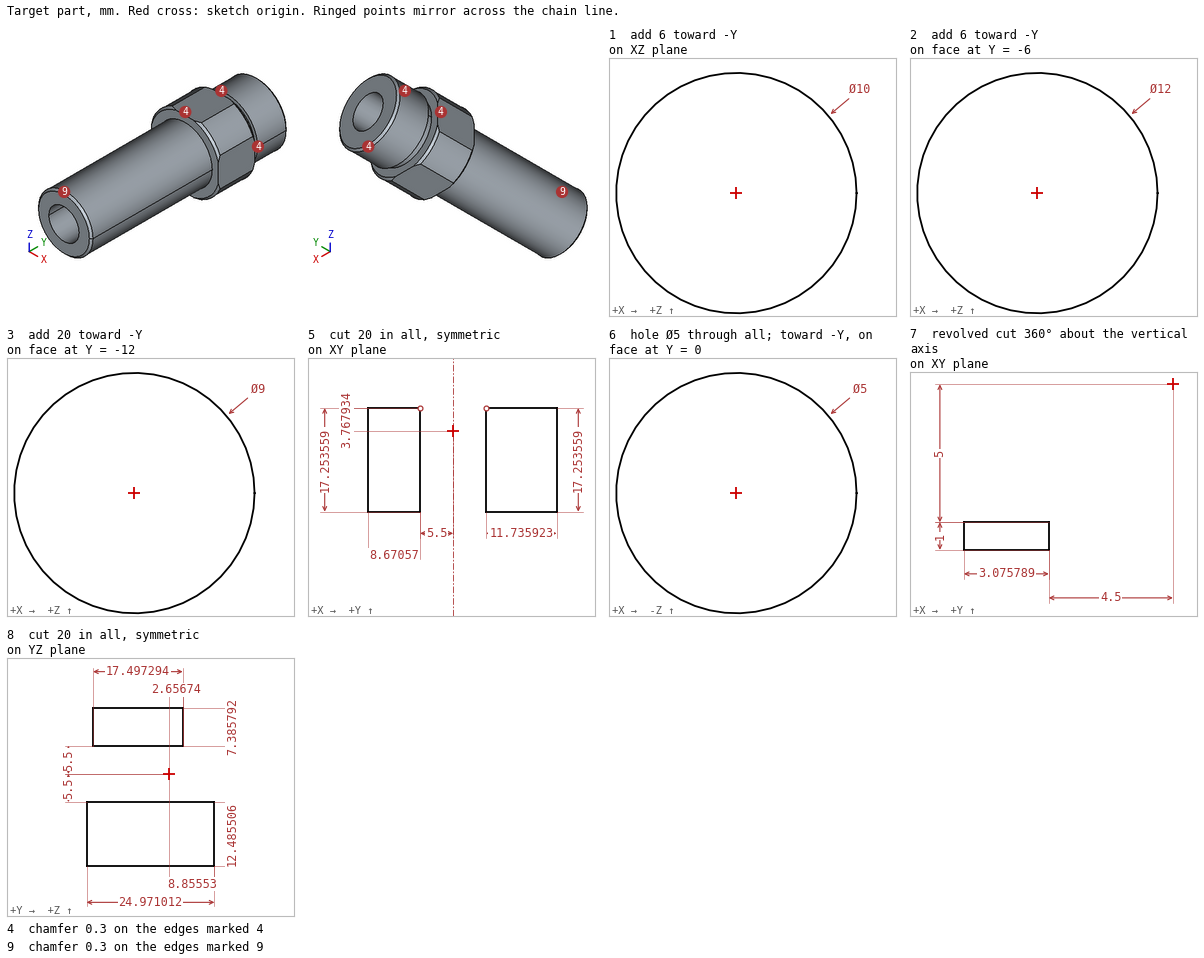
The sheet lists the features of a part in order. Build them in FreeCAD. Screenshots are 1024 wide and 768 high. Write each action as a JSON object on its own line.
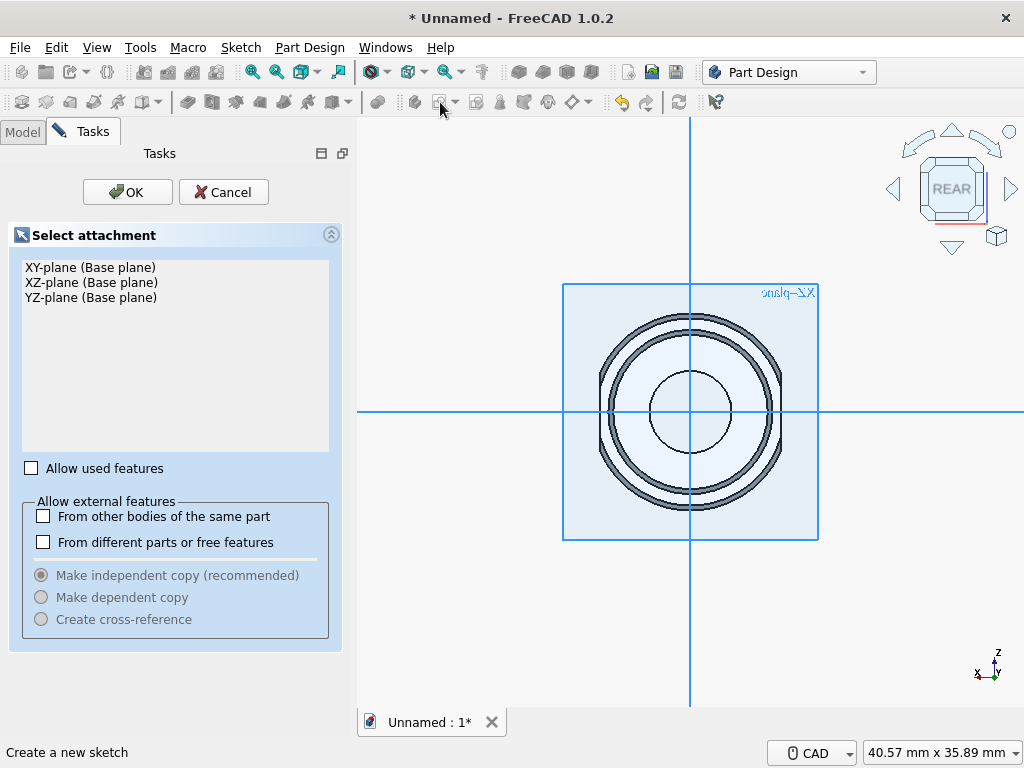
{"action": "left_click", "coordinate": [82, 268]}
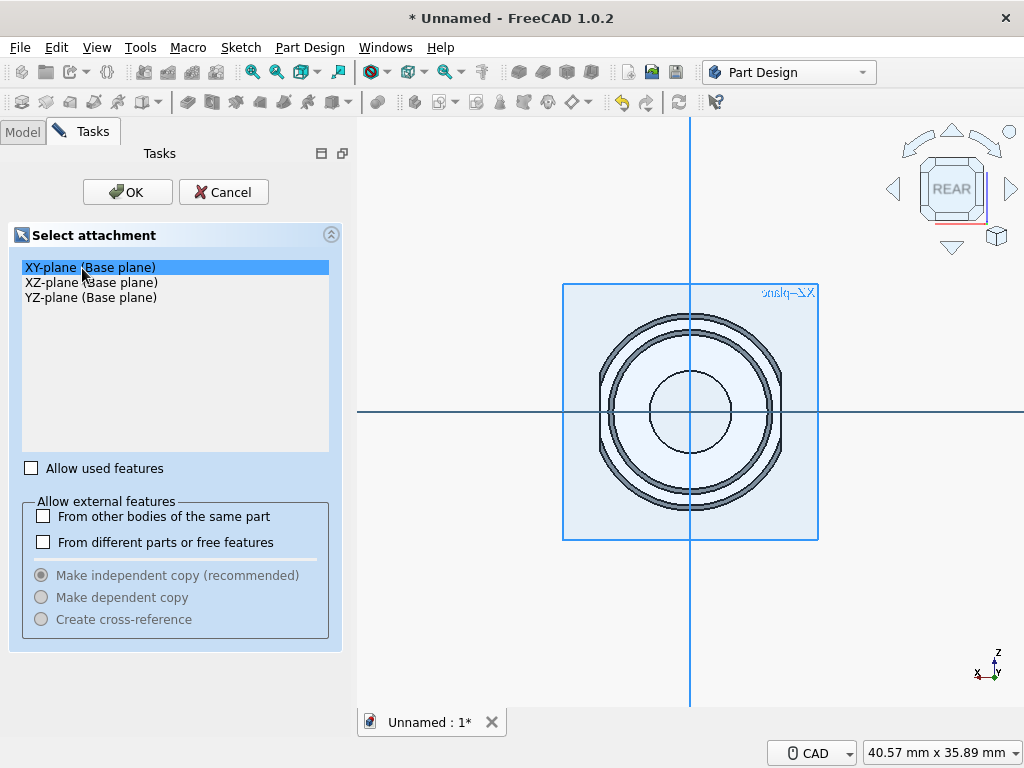
{"action": "left_click", "coordinate": [128, 192]}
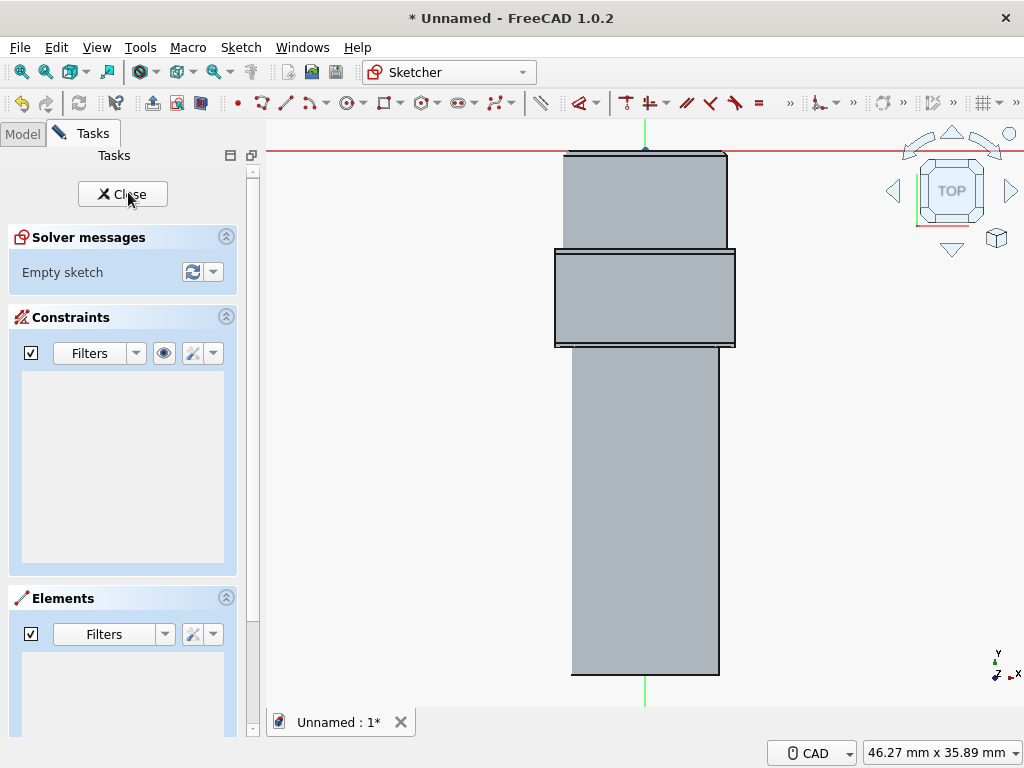
{"action": "left_click", "coordinate": [202, 104]}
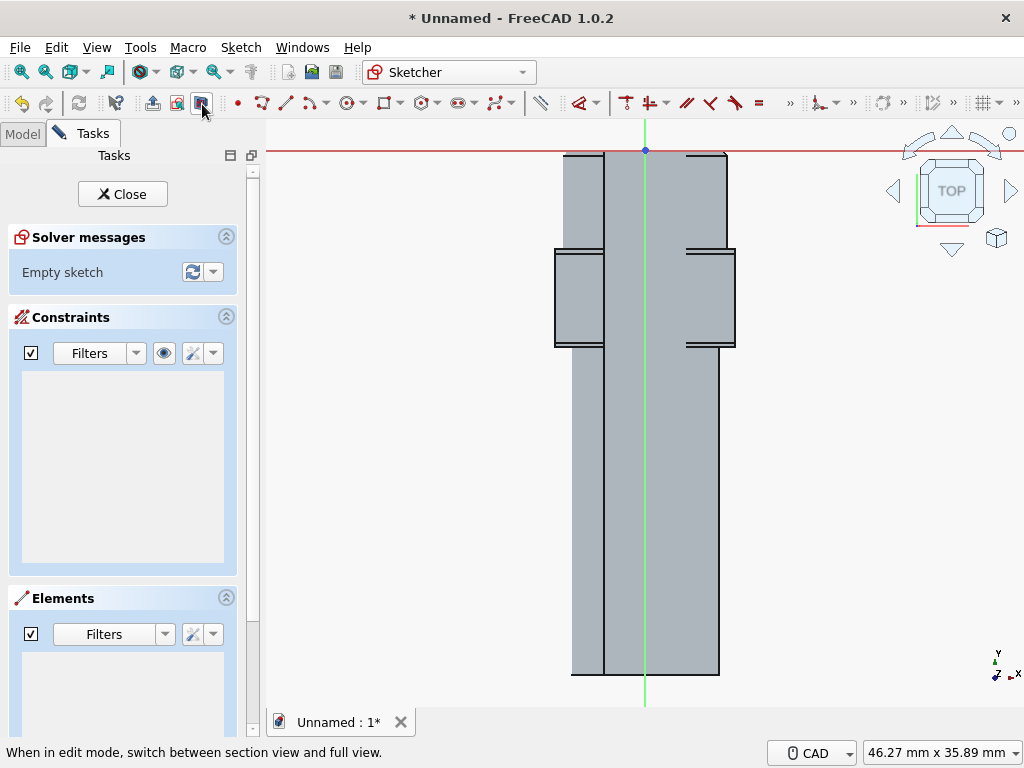
{"action": "scroll", "coordinate": [576, 413], "scroll_direction": "down", "scroll_amount": 5}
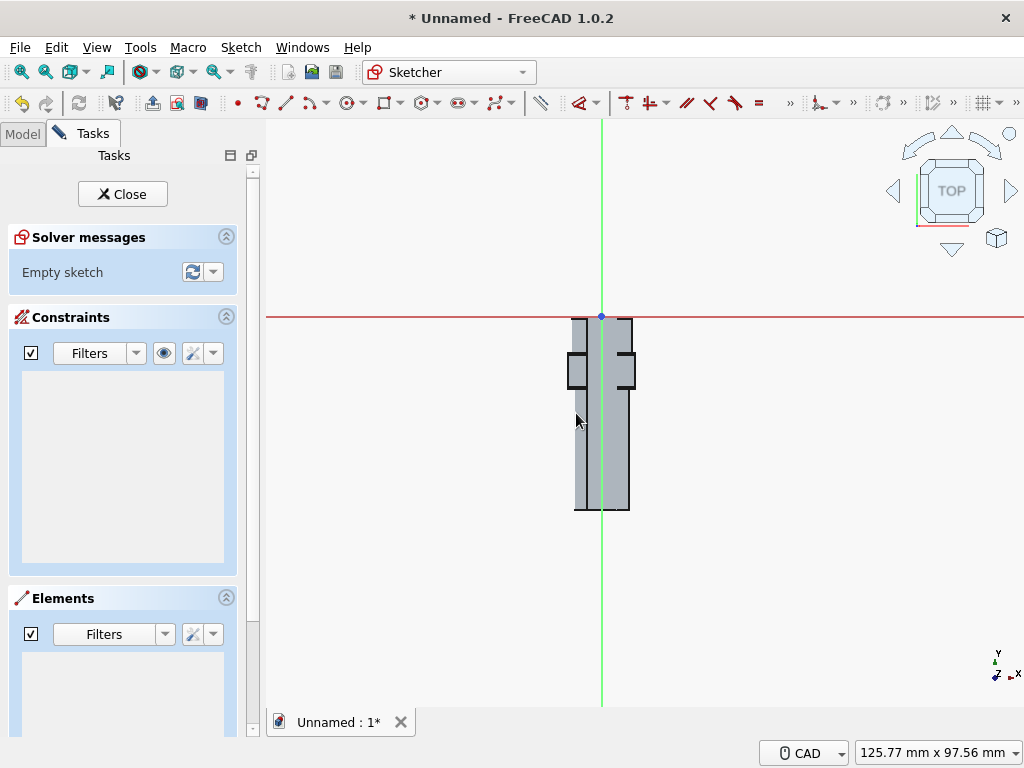
{"action": "scroll", "coordinate": [579, 325], "scroll_direction": "up", "scroll_amount": 11}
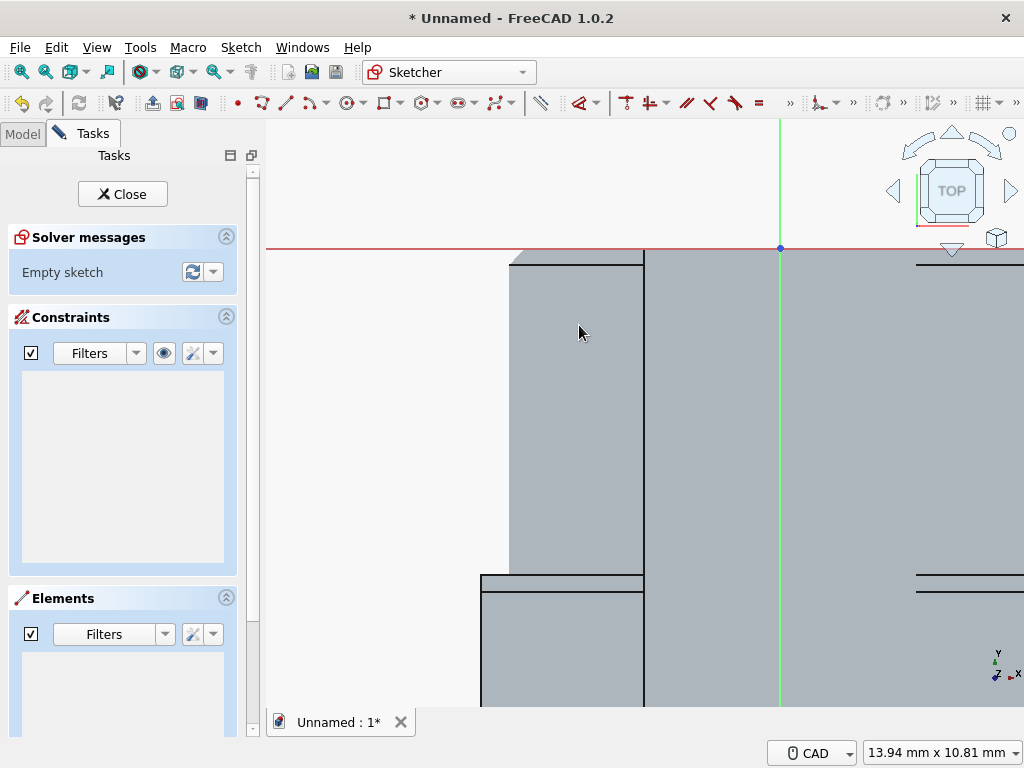
{"action": "key", "text": "g r"}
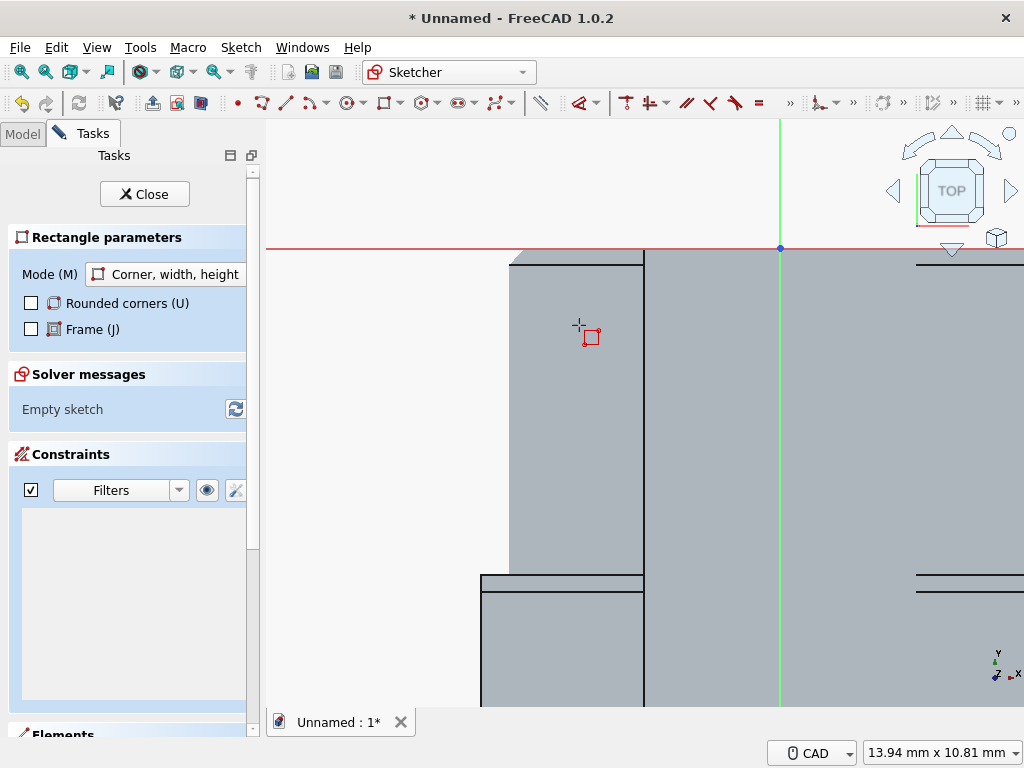
{"action": "left_click", "coordinate": [368, 521]}
{"action": "mouse_move", "coordinate": [535, 575]}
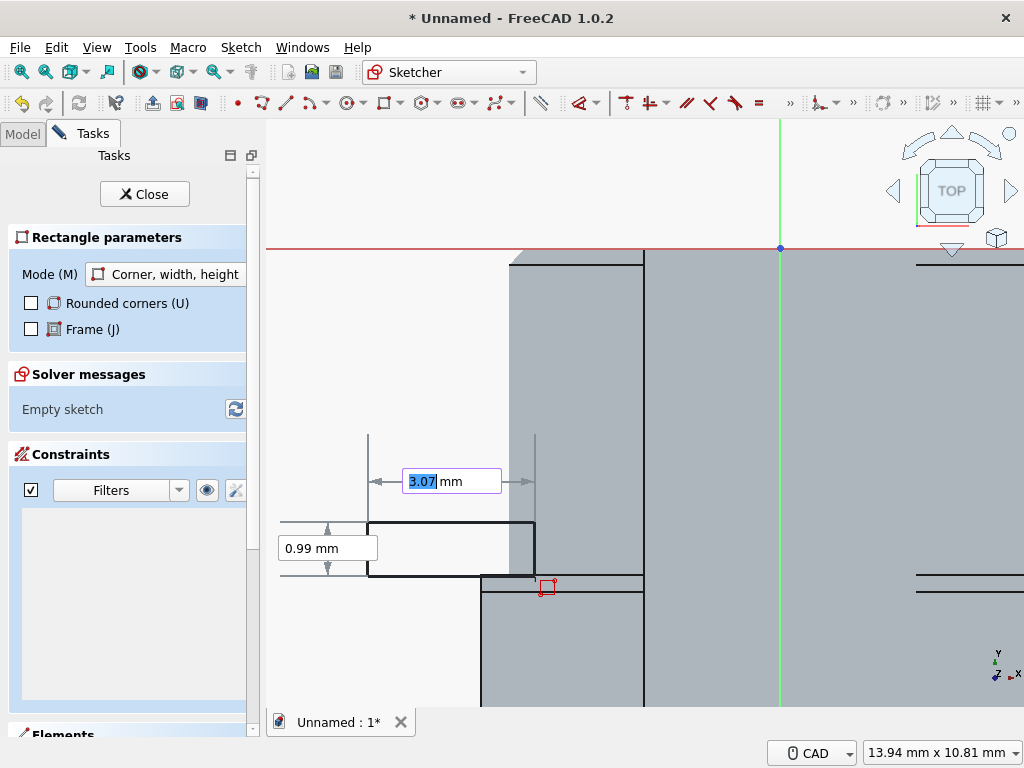
{"action": "type", "text": "3.075789"}
{"action": "key", "text": "Tab"}
{"action": "type", "text": "1"}
{"action": "key", "text": "Return"}
{"action": "key", "text": "Escape"}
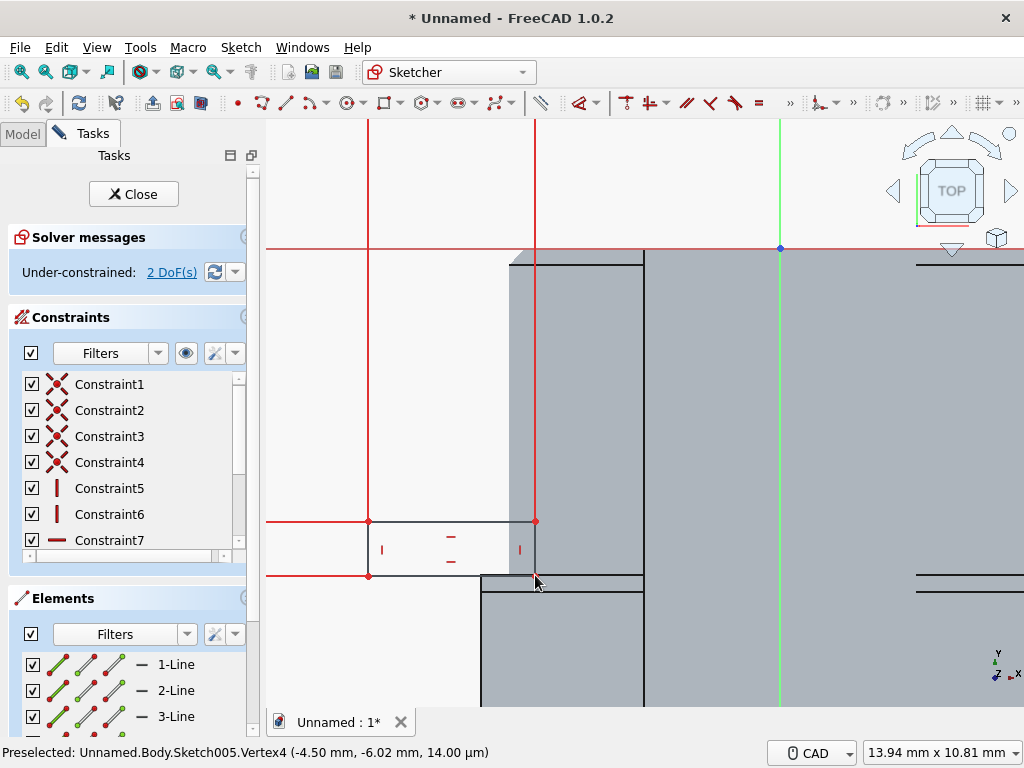
{"action": "key", "text": "d"}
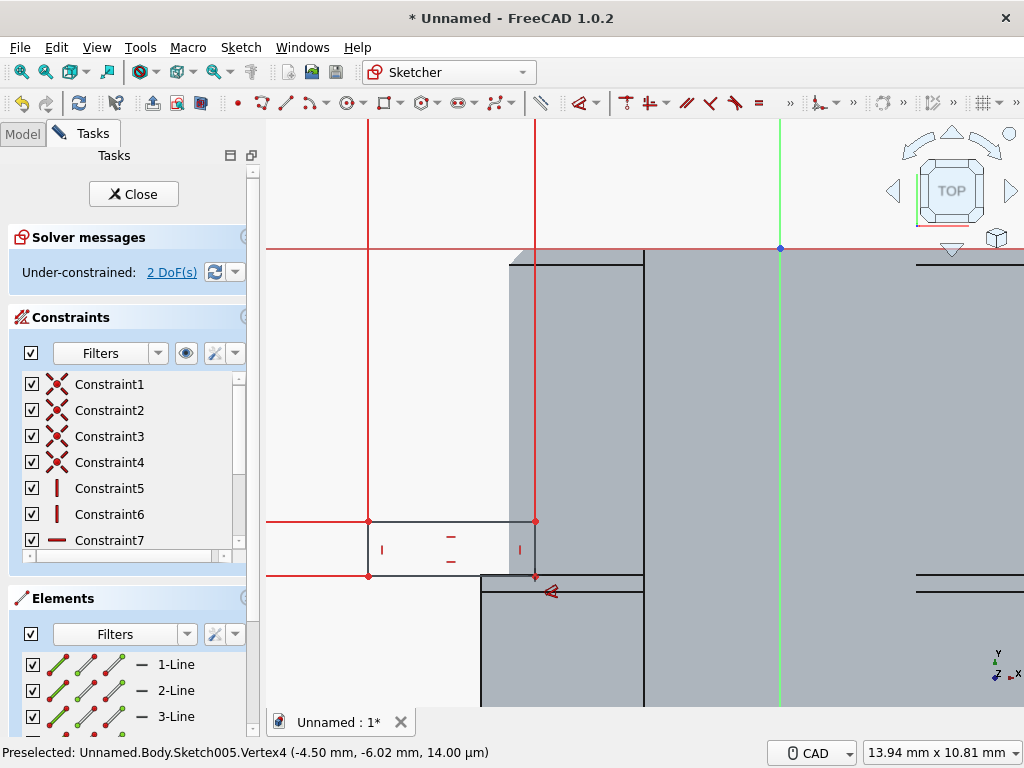
{"action": "left_click", "coordinate": [368, 522]}
{"action": "left_click", "coordinate": [814, 385]}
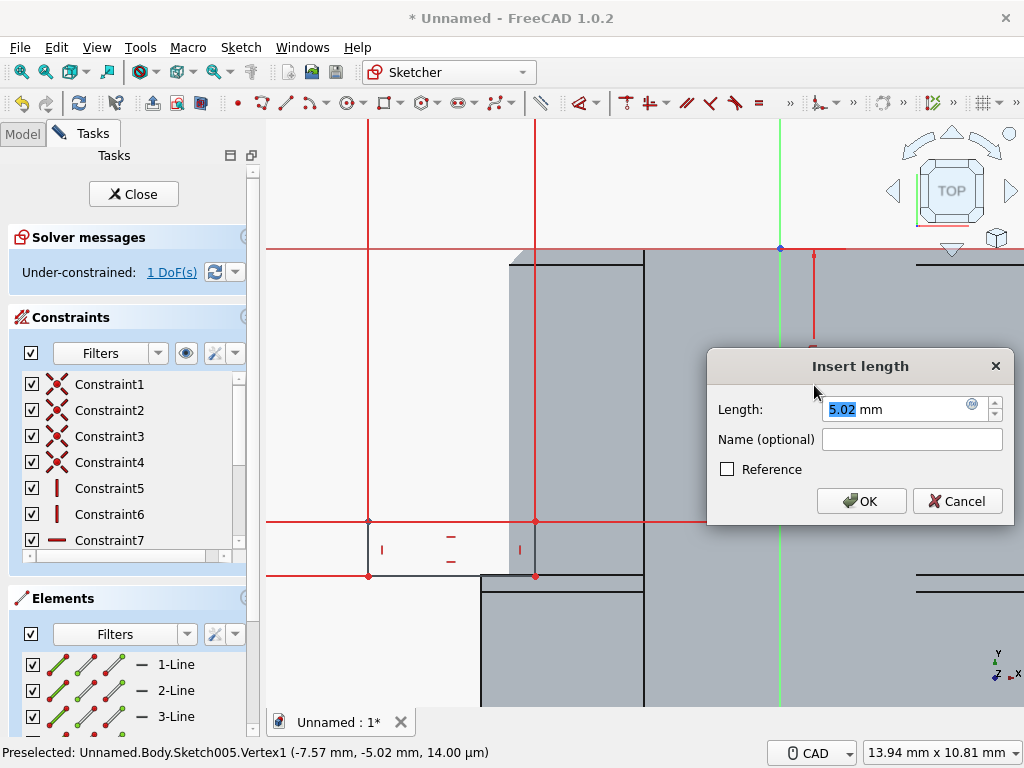
{"action": "type", "text": "5"}
{"action": "key", "text": "Return"}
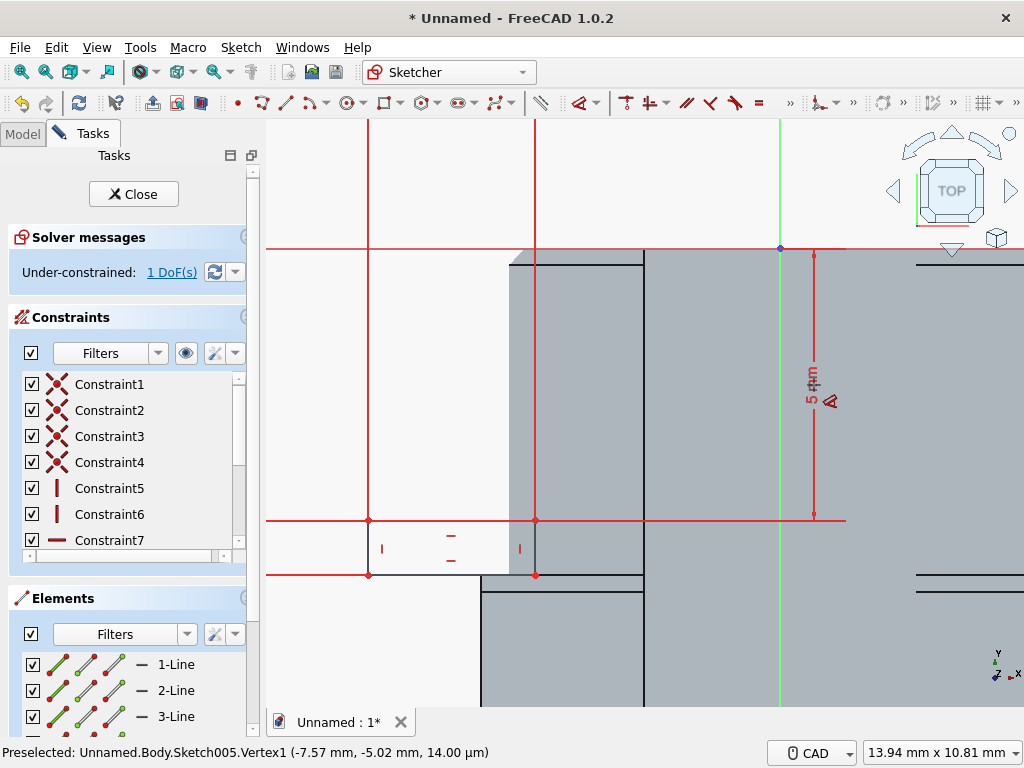
{"action": "left_click", "coordinate": [535, 575]}
{"action": "left_click", "coordinate": [658, 609]}